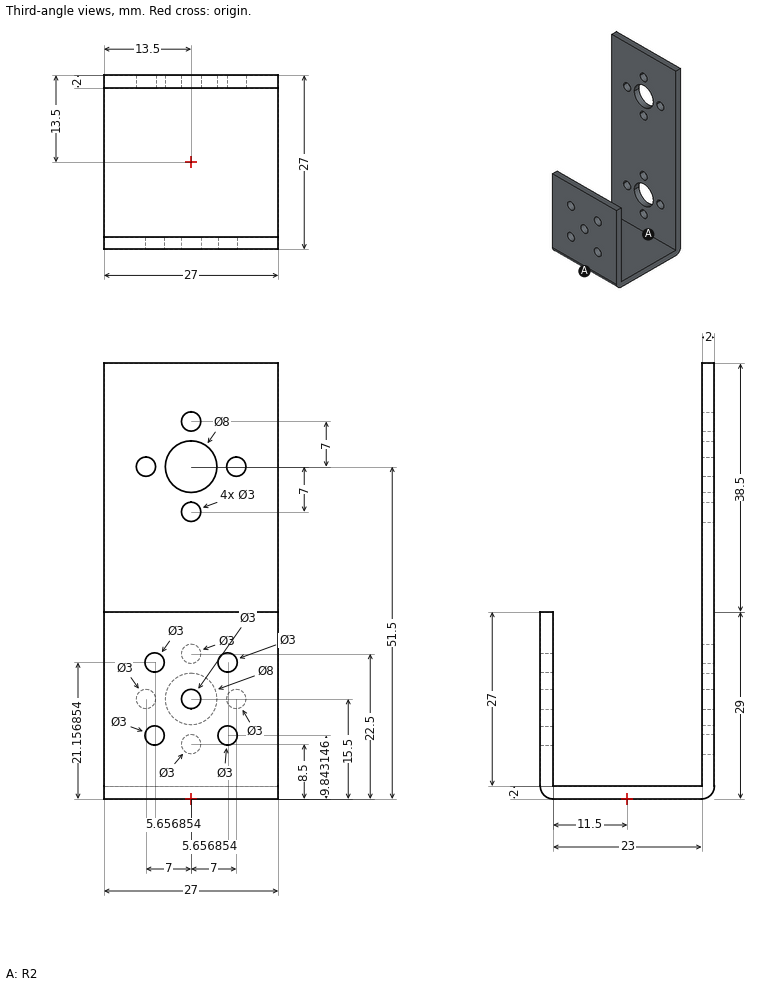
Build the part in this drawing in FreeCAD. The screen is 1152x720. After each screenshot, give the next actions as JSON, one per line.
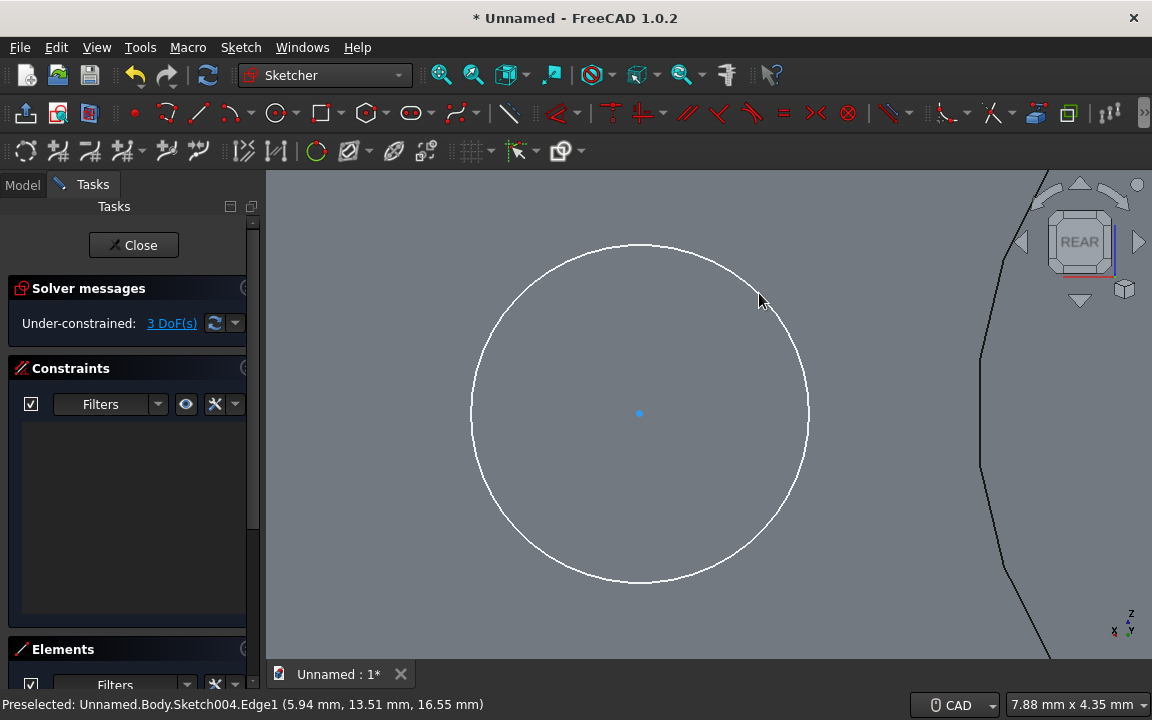
{"action": "key", "text": "d"}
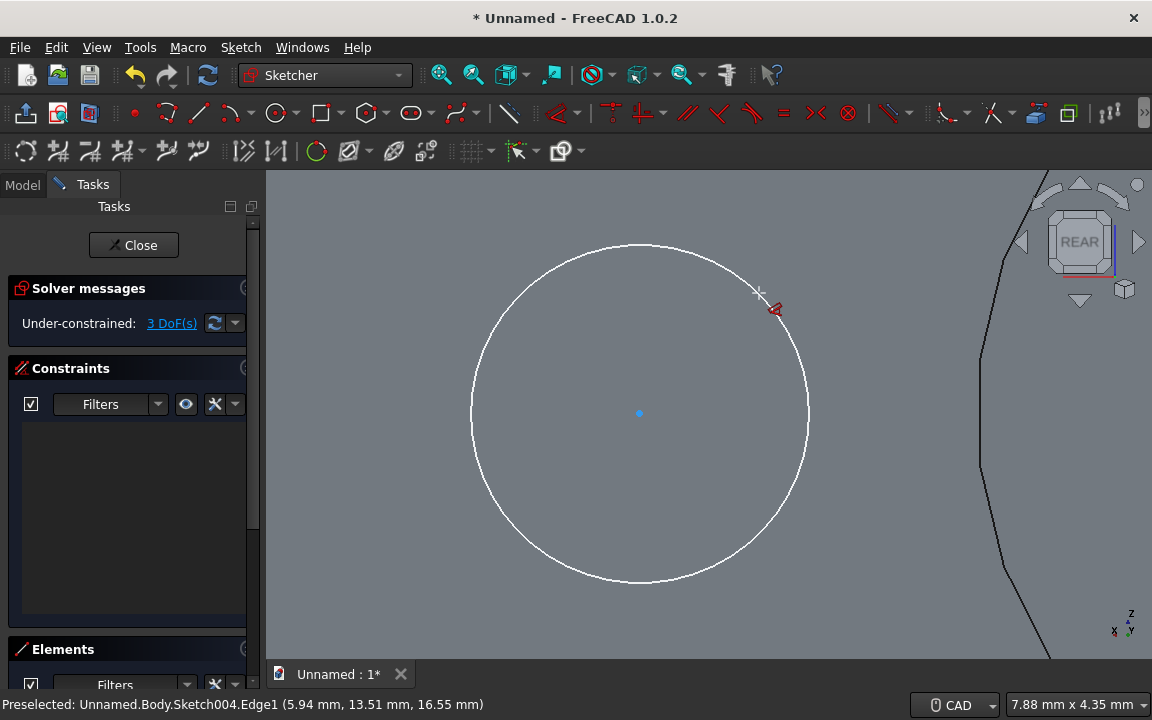
{"action": "left_click", "coordinate": [759, 294]}
{"action": "left_click", "coordinate": [782, 271]}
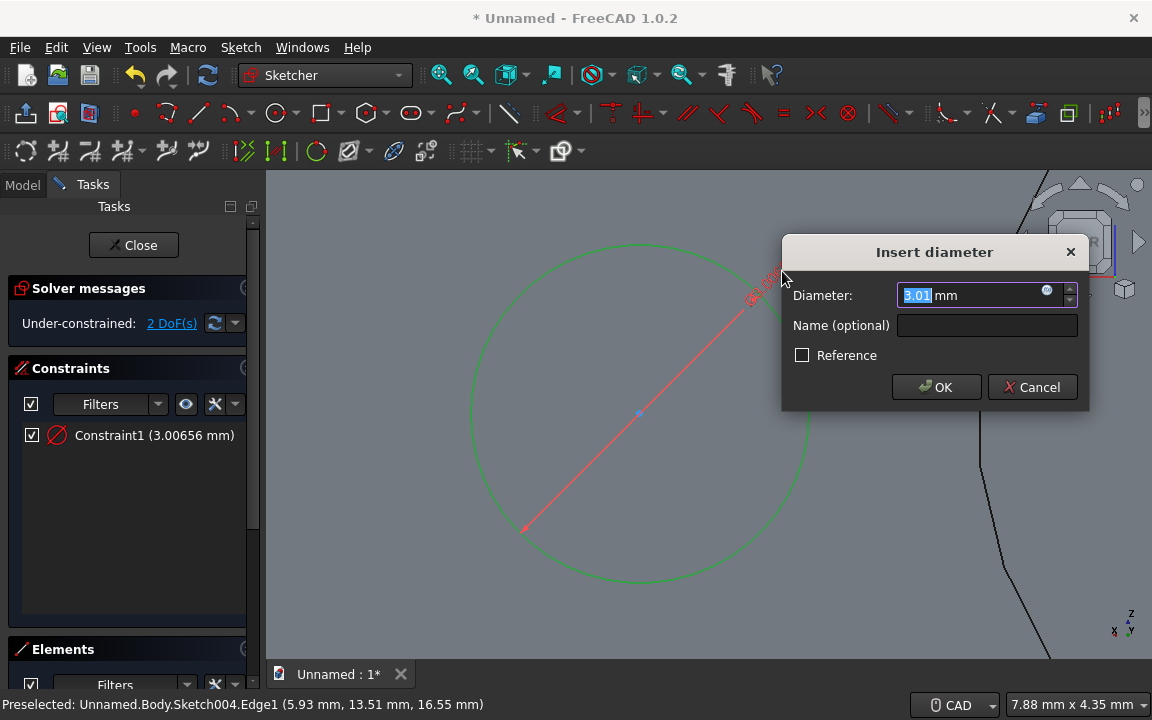
{"action": "type", "text": "3"}
{"action": "key", "text": "Return"}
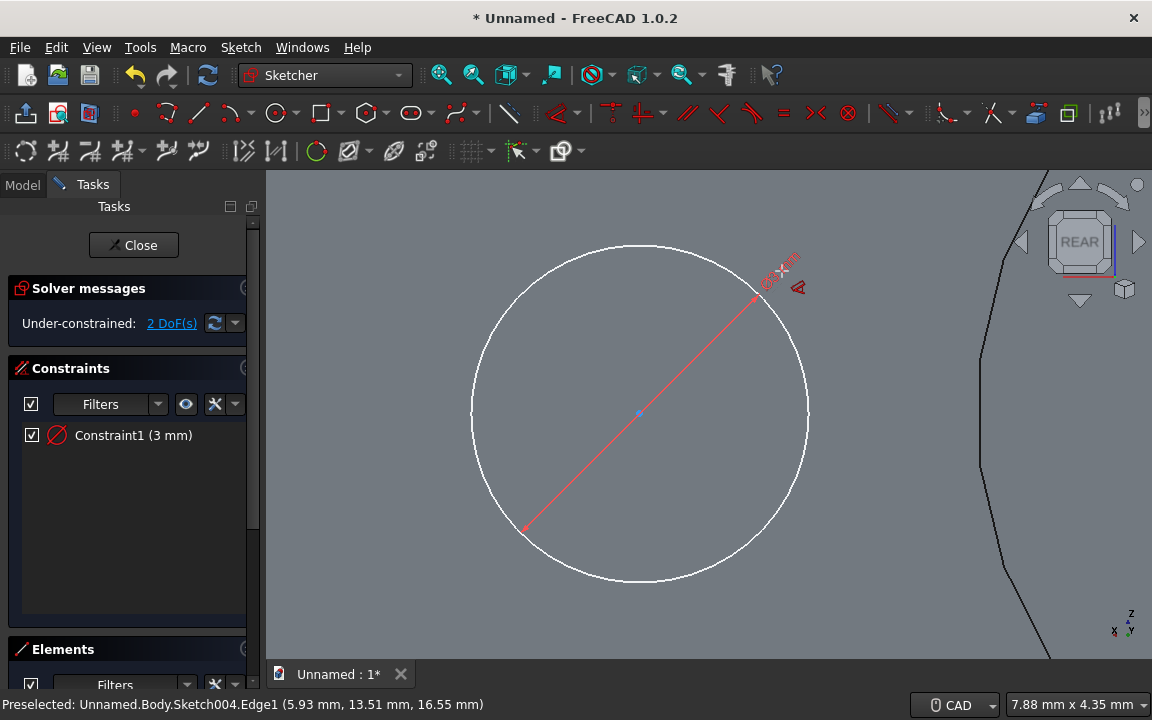
{"action": "left_click", "coordinate": [640, 414]}
{"action": "left_click", "coordinate": [734, 380]}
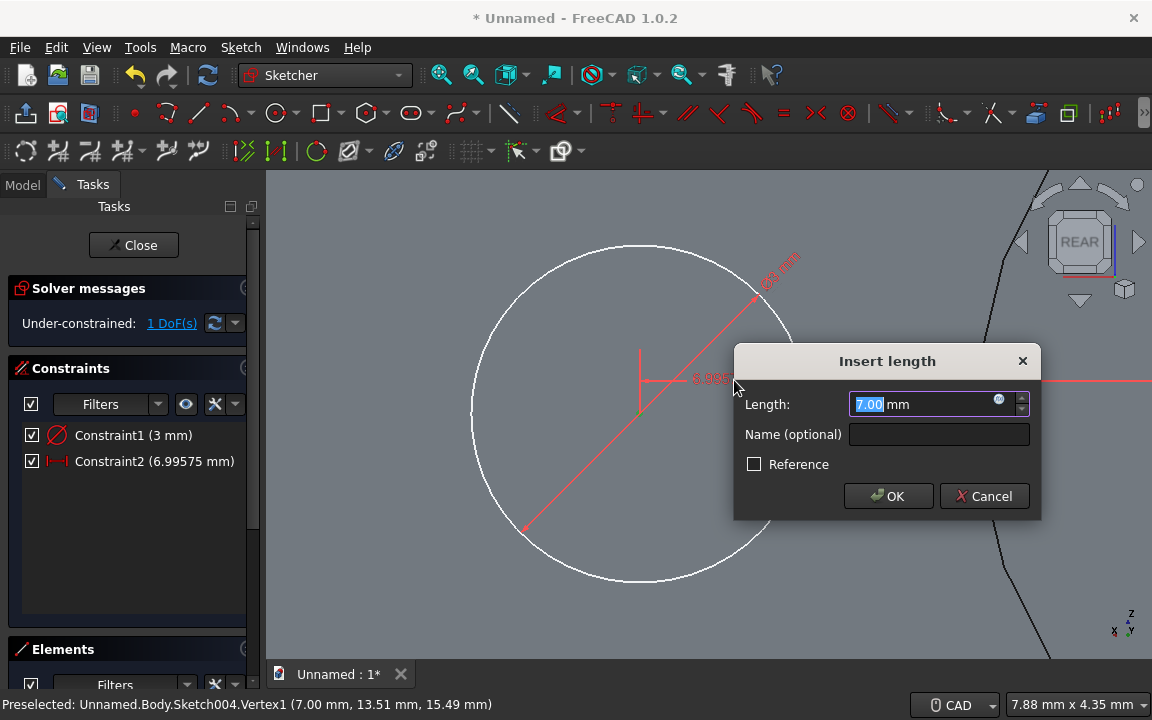
{"action": "type", "text": "7"}
{"action": "key", "text": "Return"}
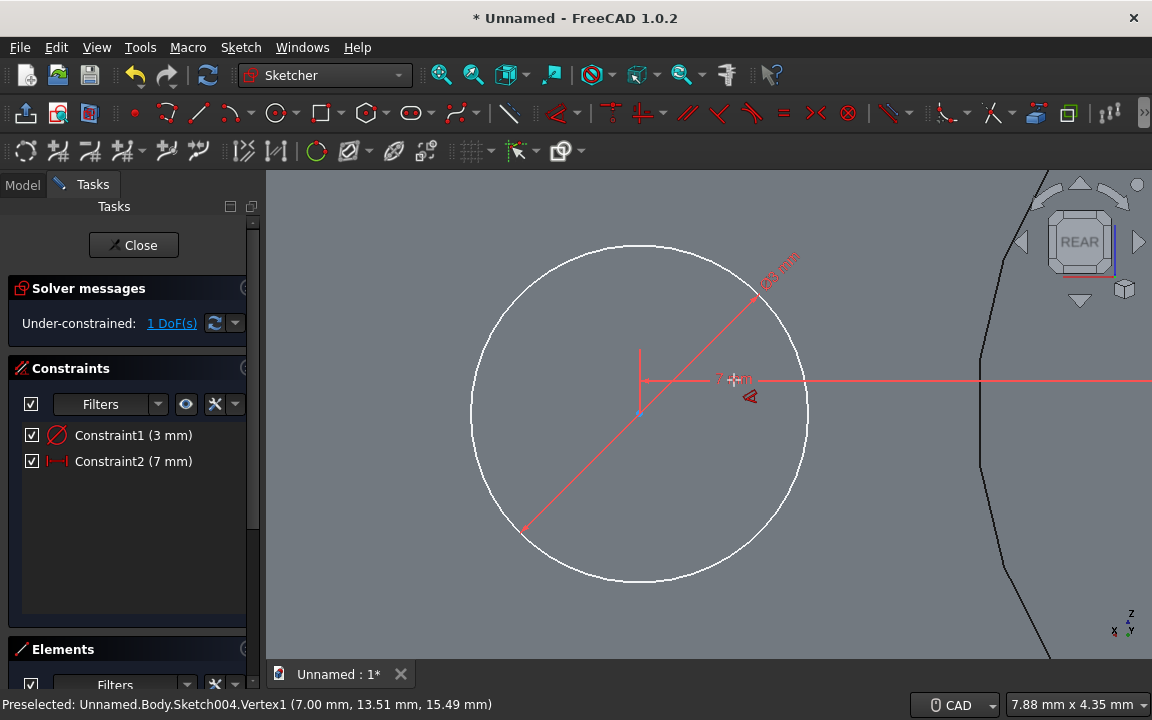
{"action": "left_click", "coordinate": [640, 414]}
{"action": "left_click", "coordinate": [606, 522]}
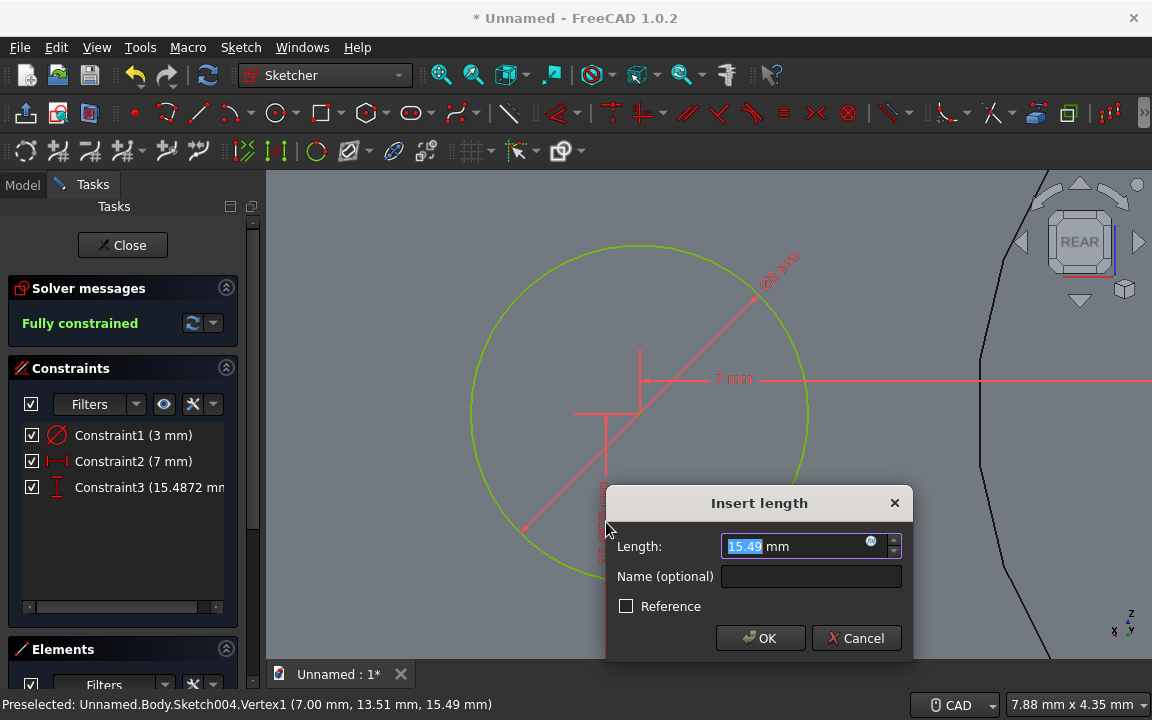
{"action": "type", "text": "15.5"}
{"action": "key", "text": "Return"}
{"action": "key", "text": "Escape"}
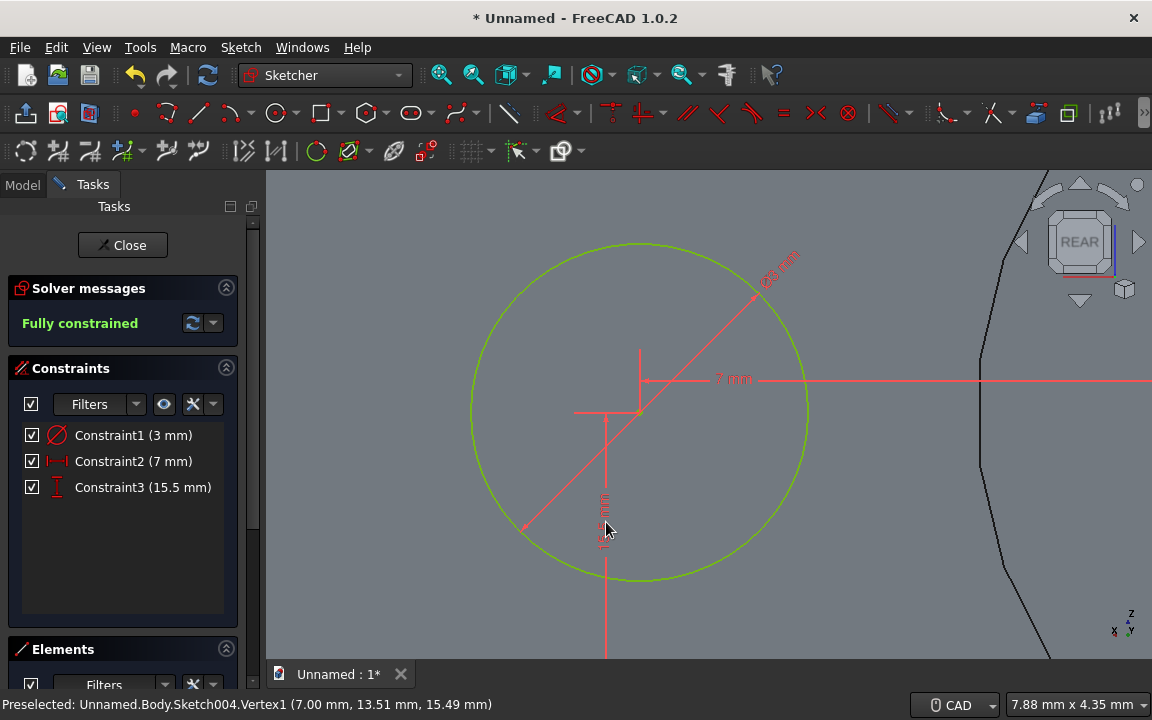
{"action": "left_click", "coordinate": [123, 245]}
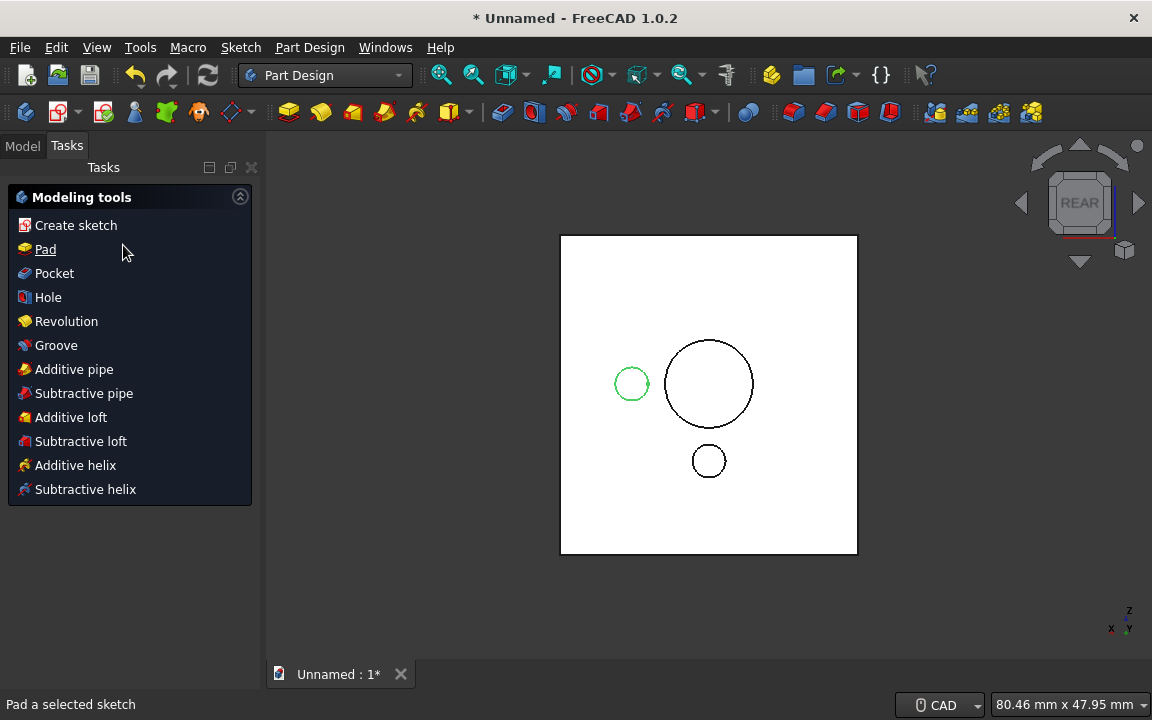
{"action": "left_click", "coordinate": [504, 112]}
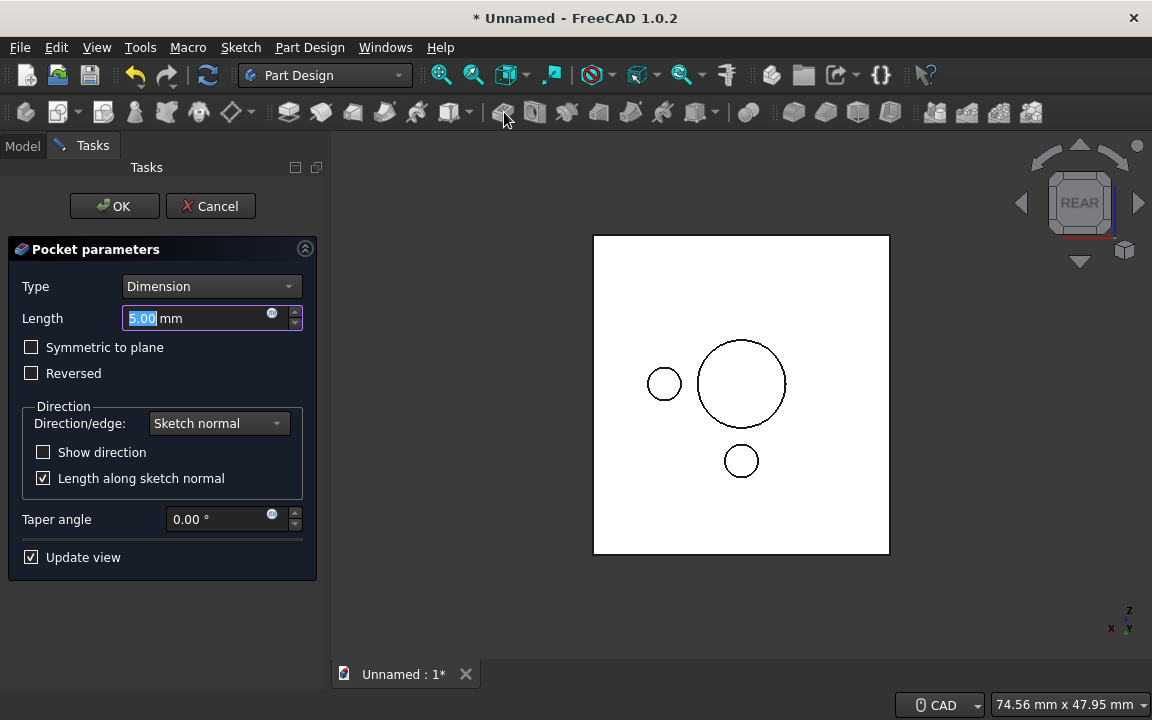
{"action": "left_click", "coordinate": [212, 286]}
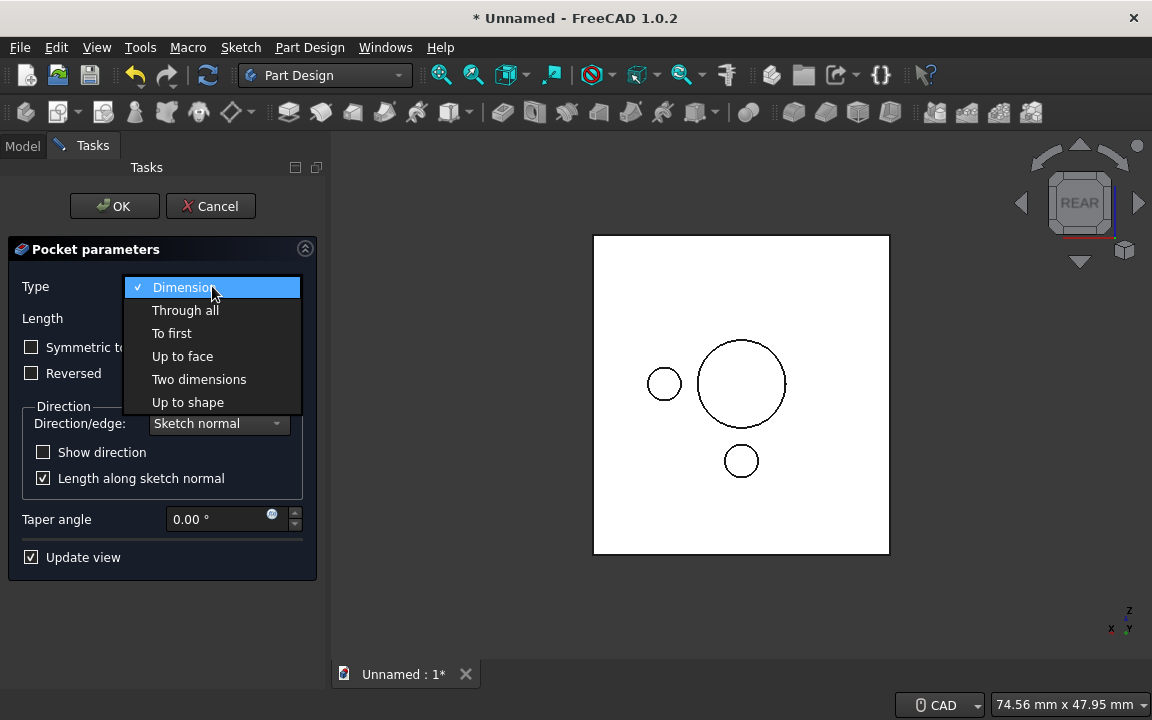
{"action": "left_click", "coordinate": [212, 334]}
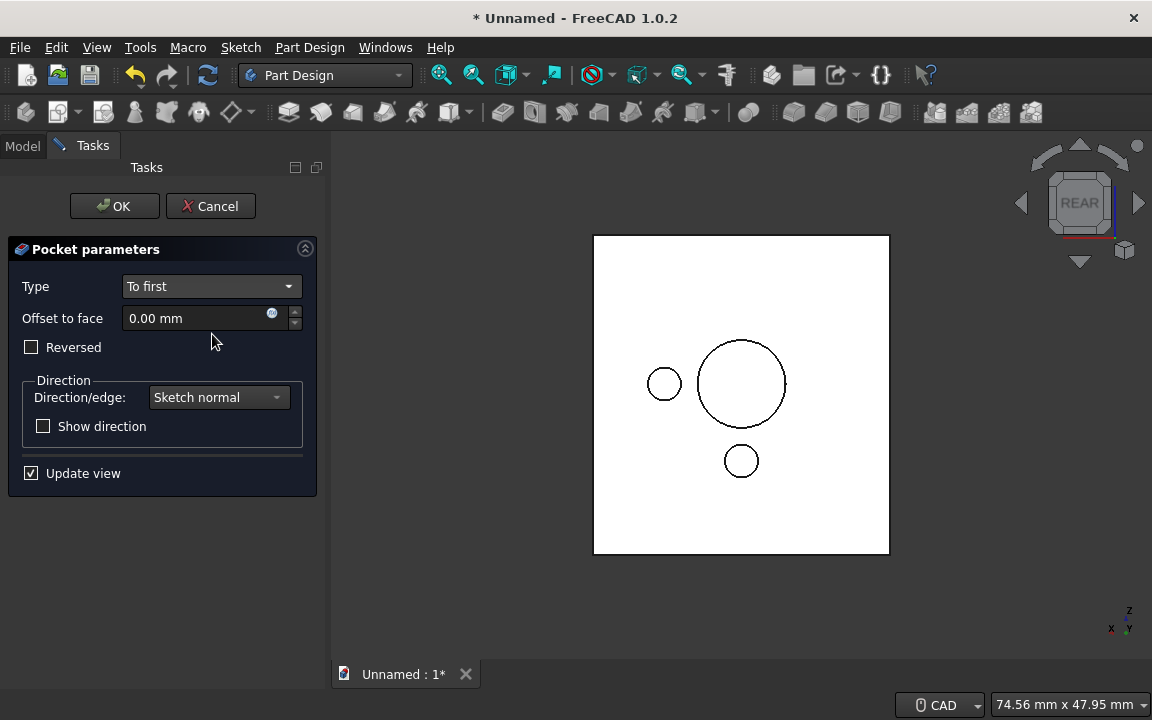
{"action": "left_click", "coordinate": [115, 206]}